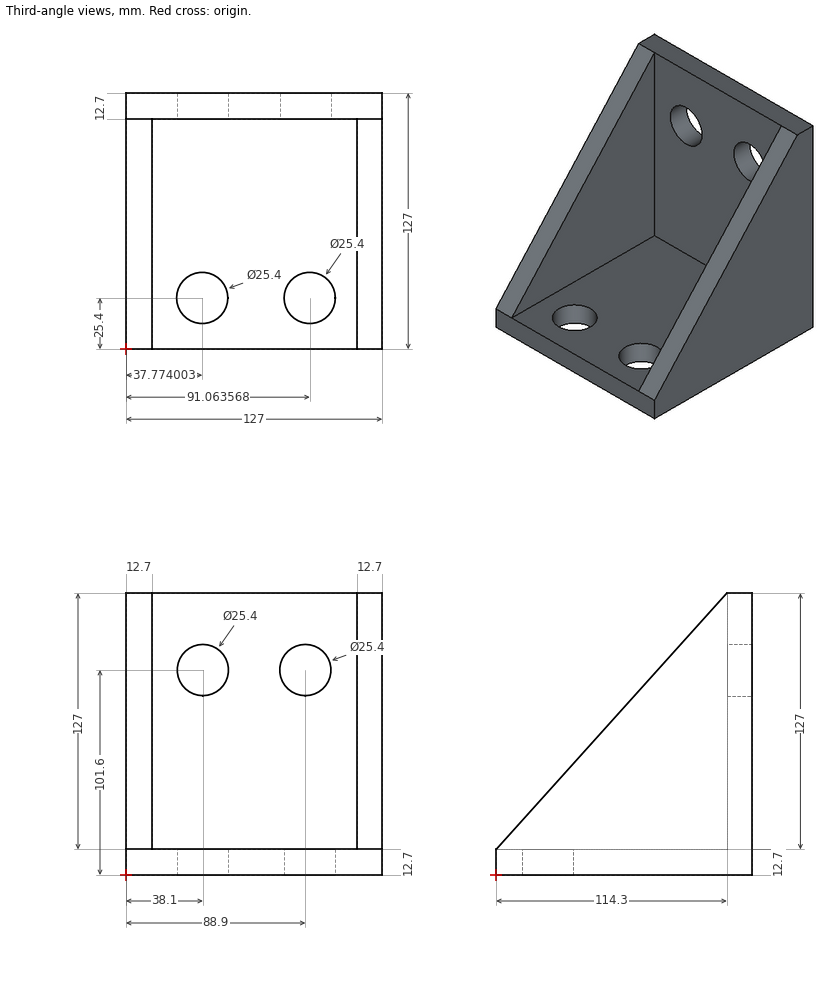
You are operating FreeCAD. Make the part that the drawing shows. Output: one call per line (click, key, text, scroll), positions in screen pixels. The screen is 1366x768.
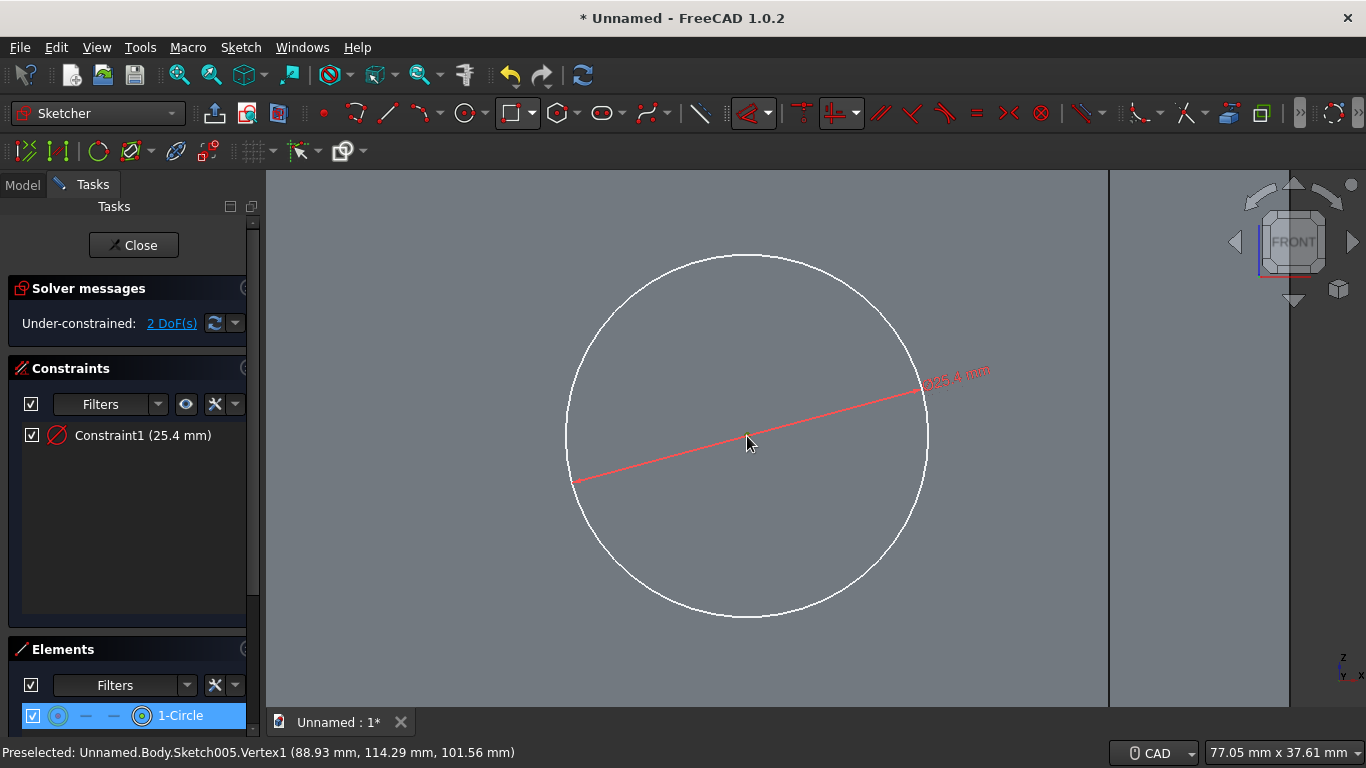
key(l)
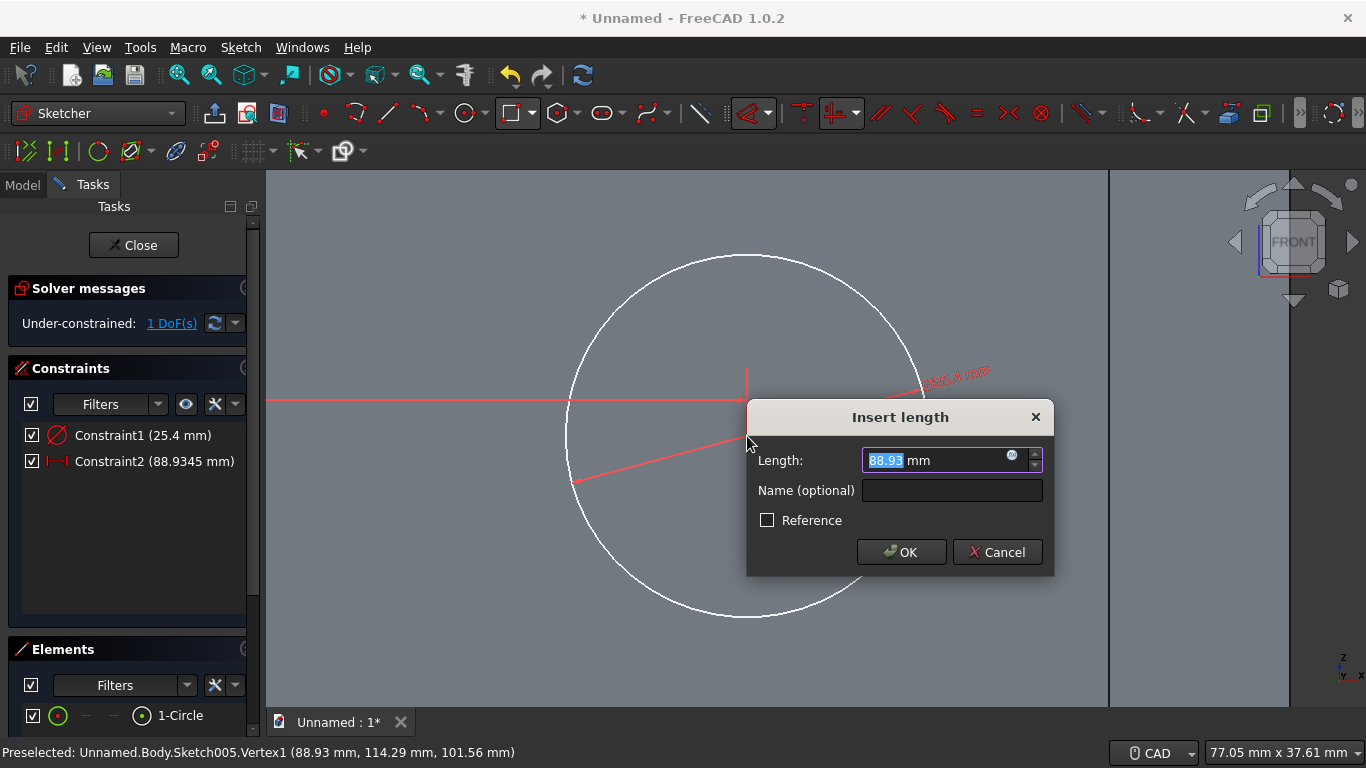
text(88.9)
key(Return)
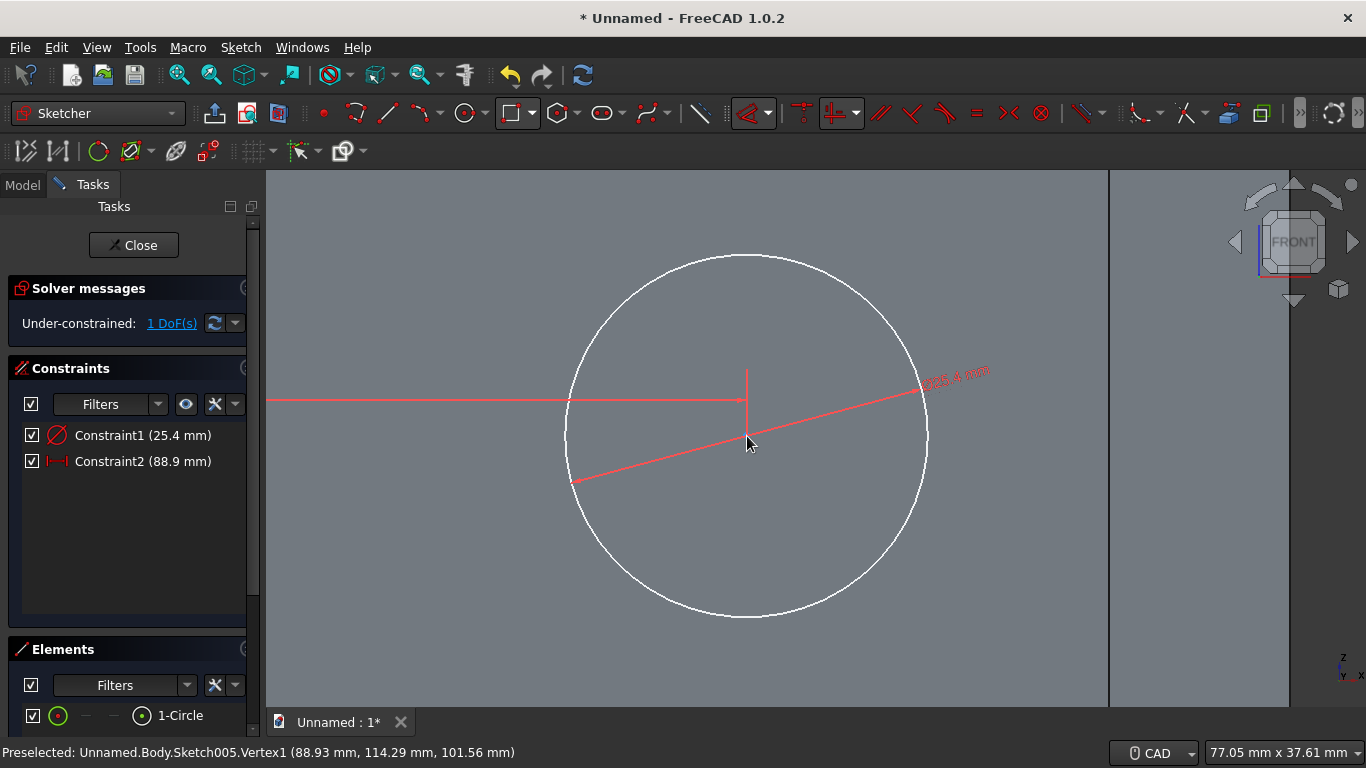
click(747, 436)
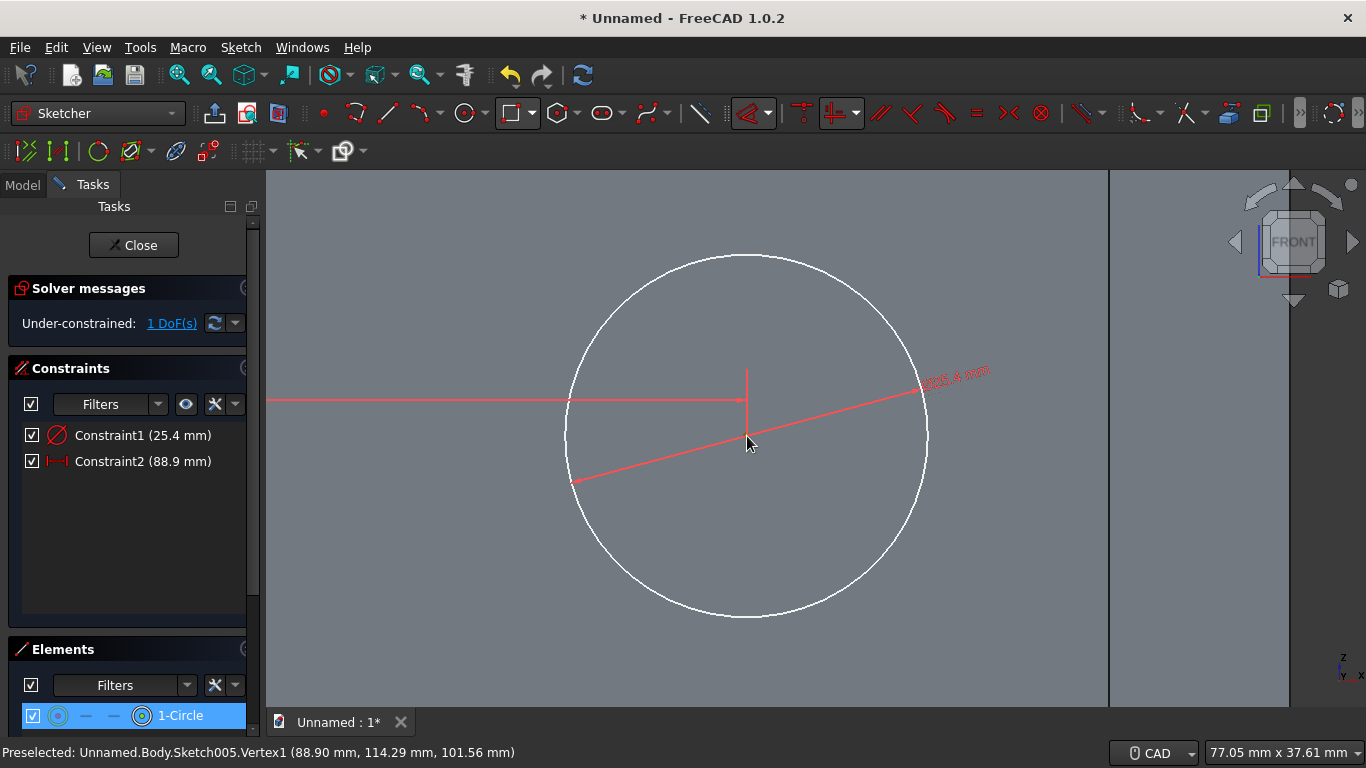
key(i)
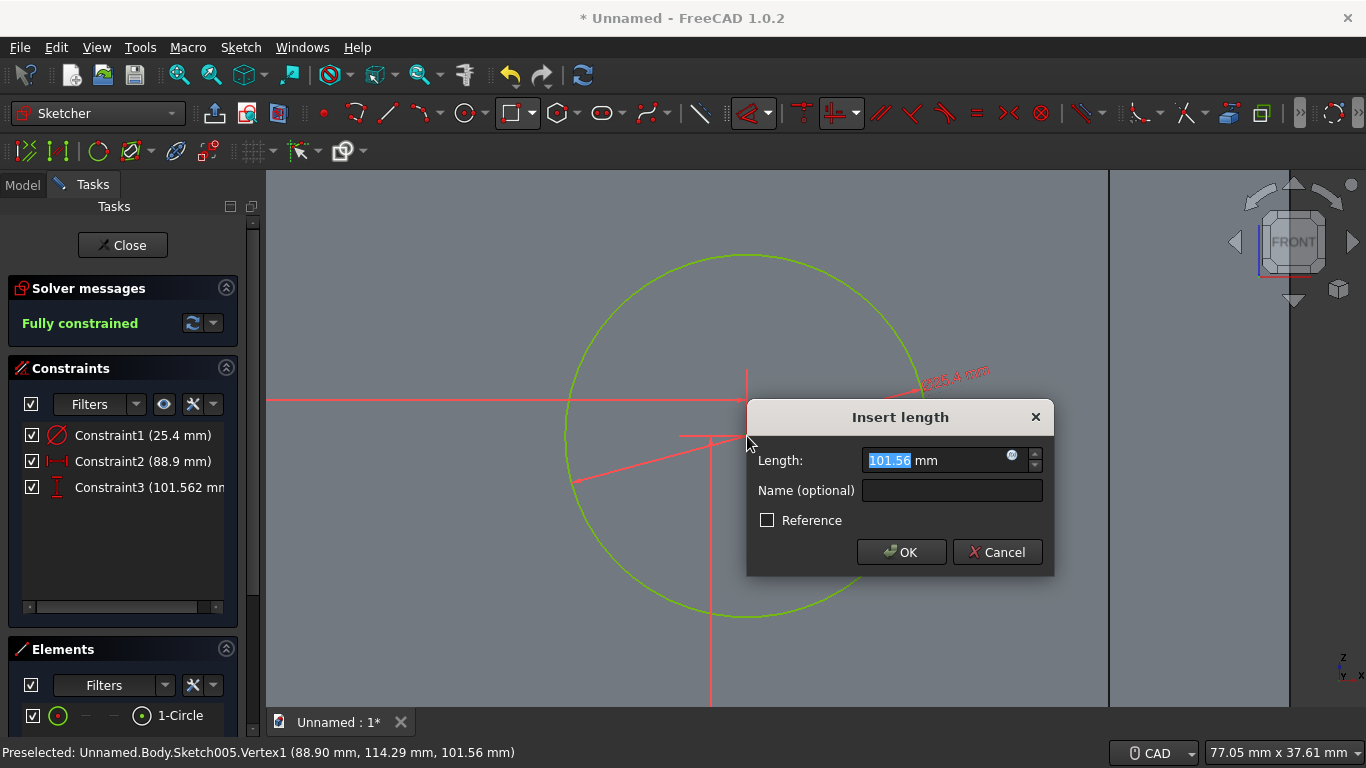
text(101.6)
key(Return)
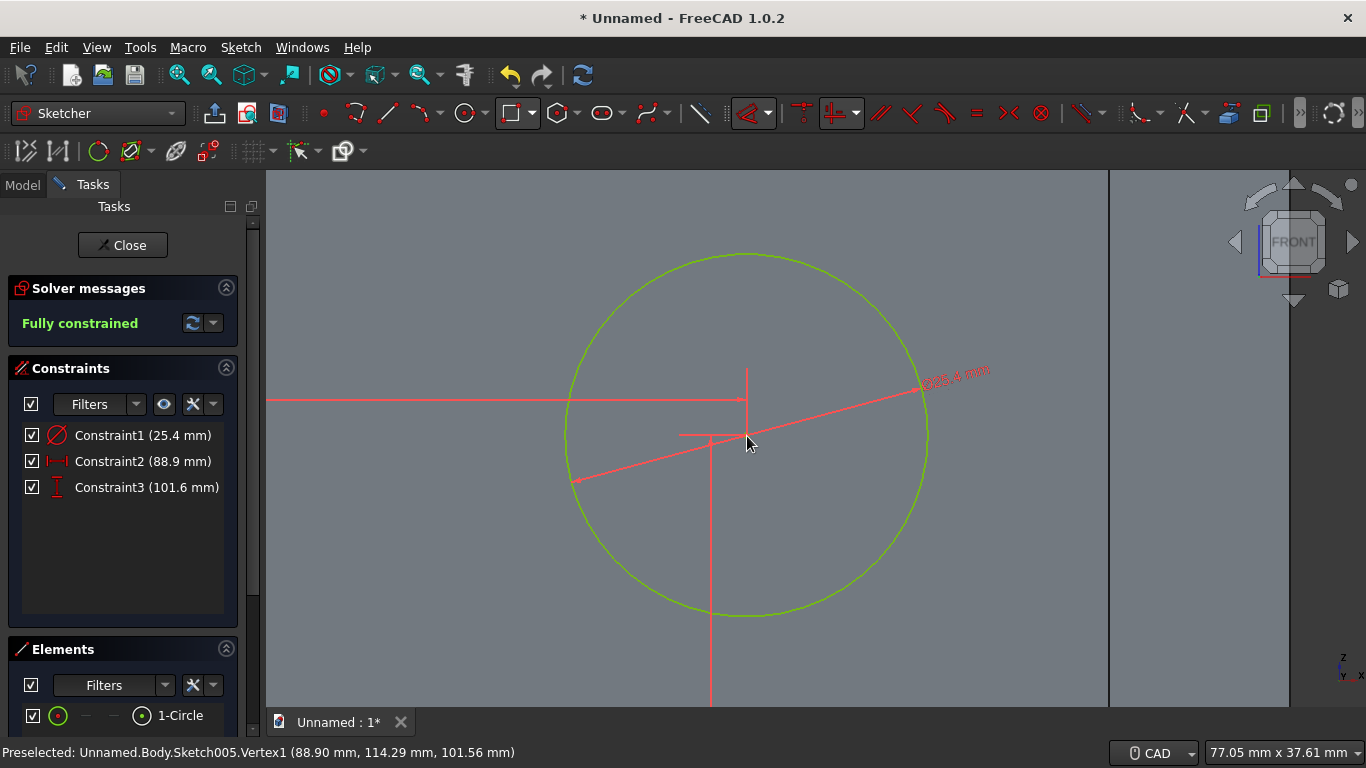
click(123, 245)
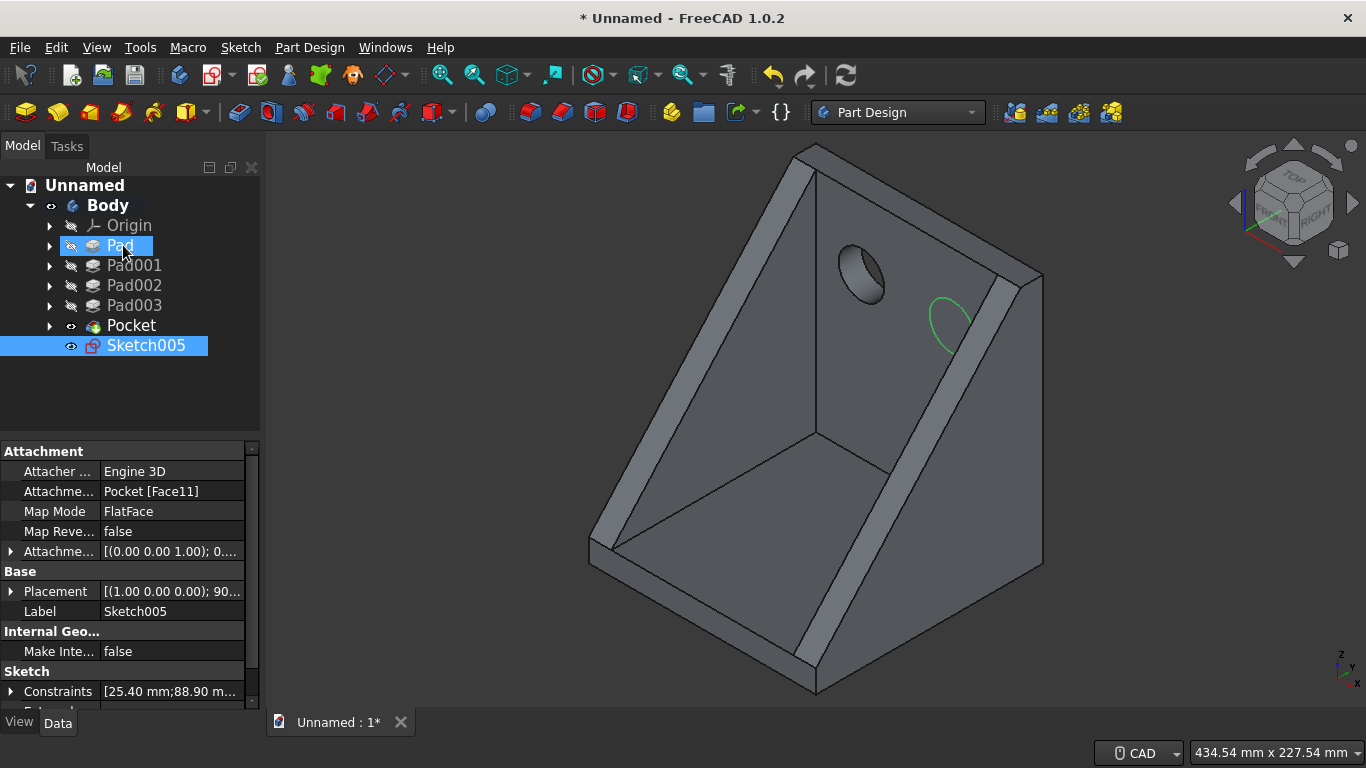
click(240, 112)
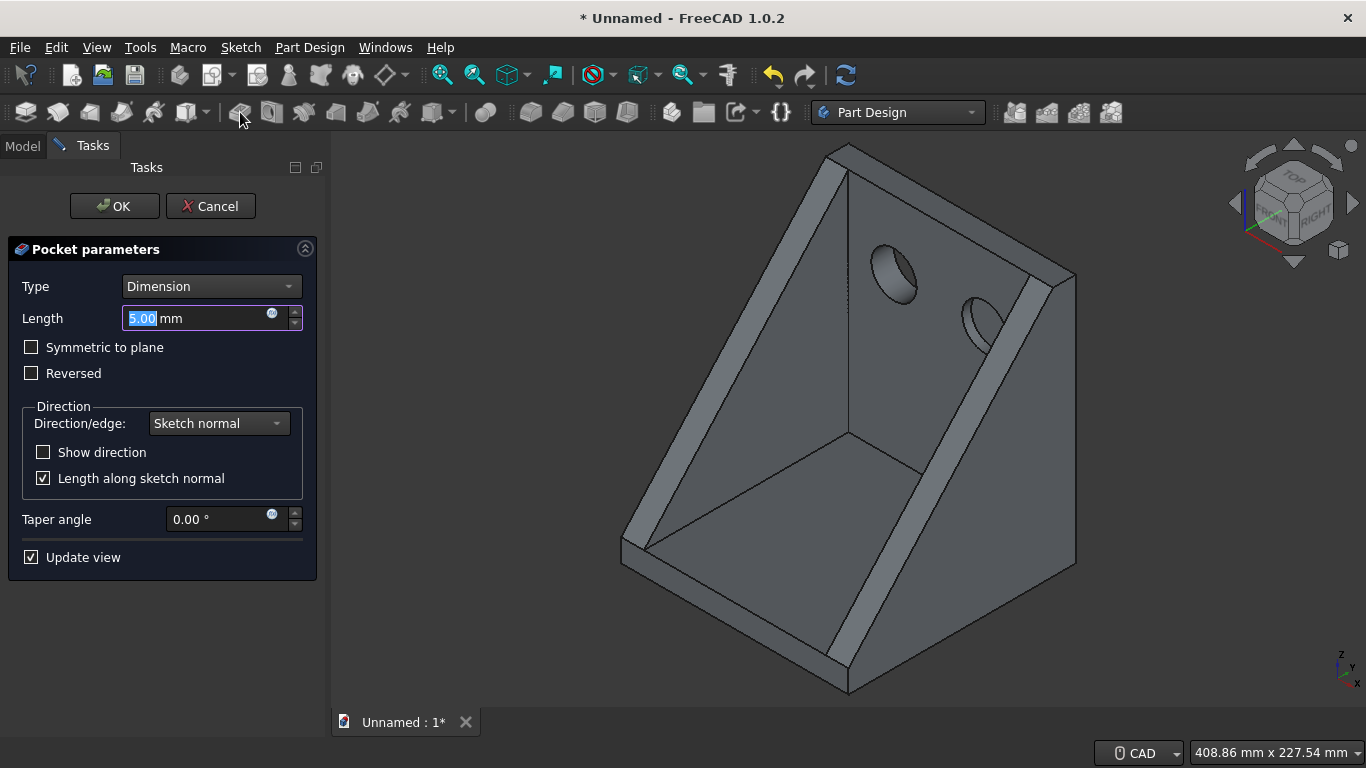
text(12.7)
key(Tab)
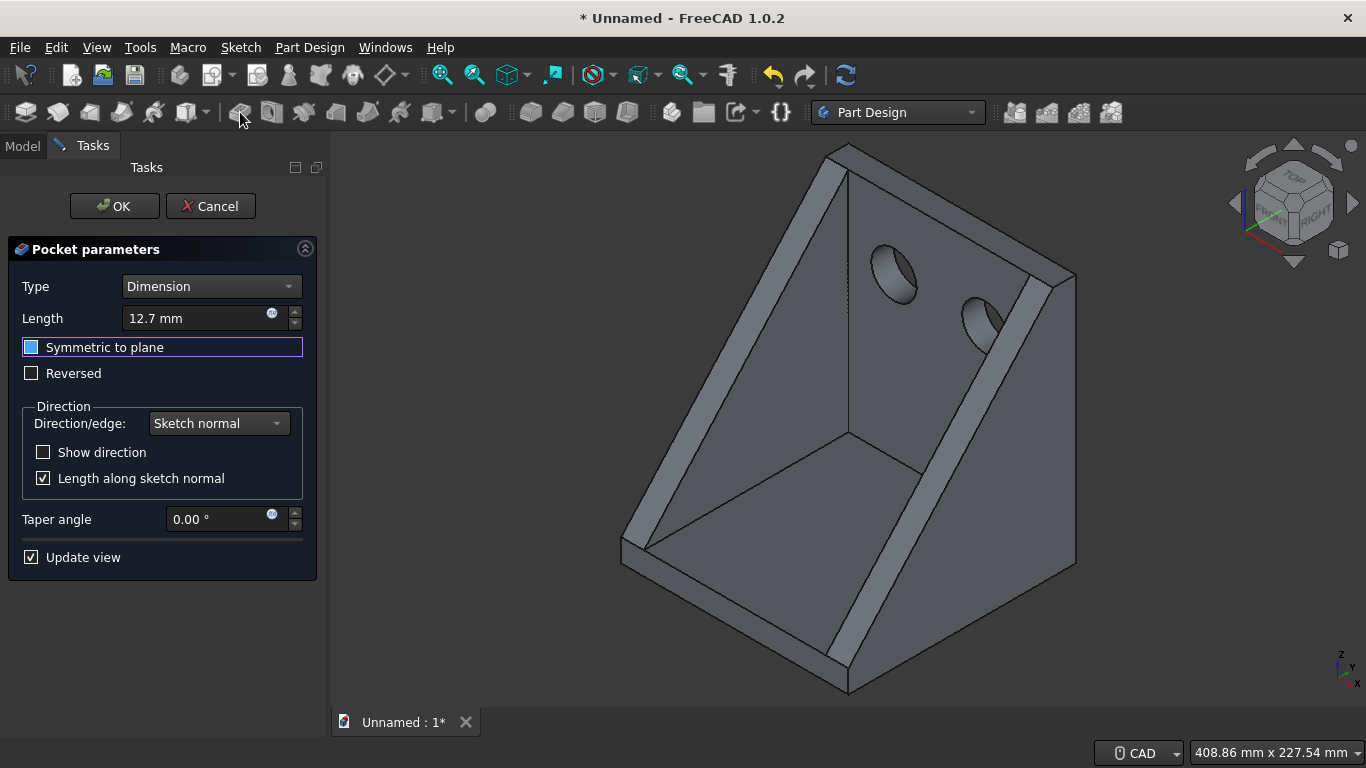
click(115, 206)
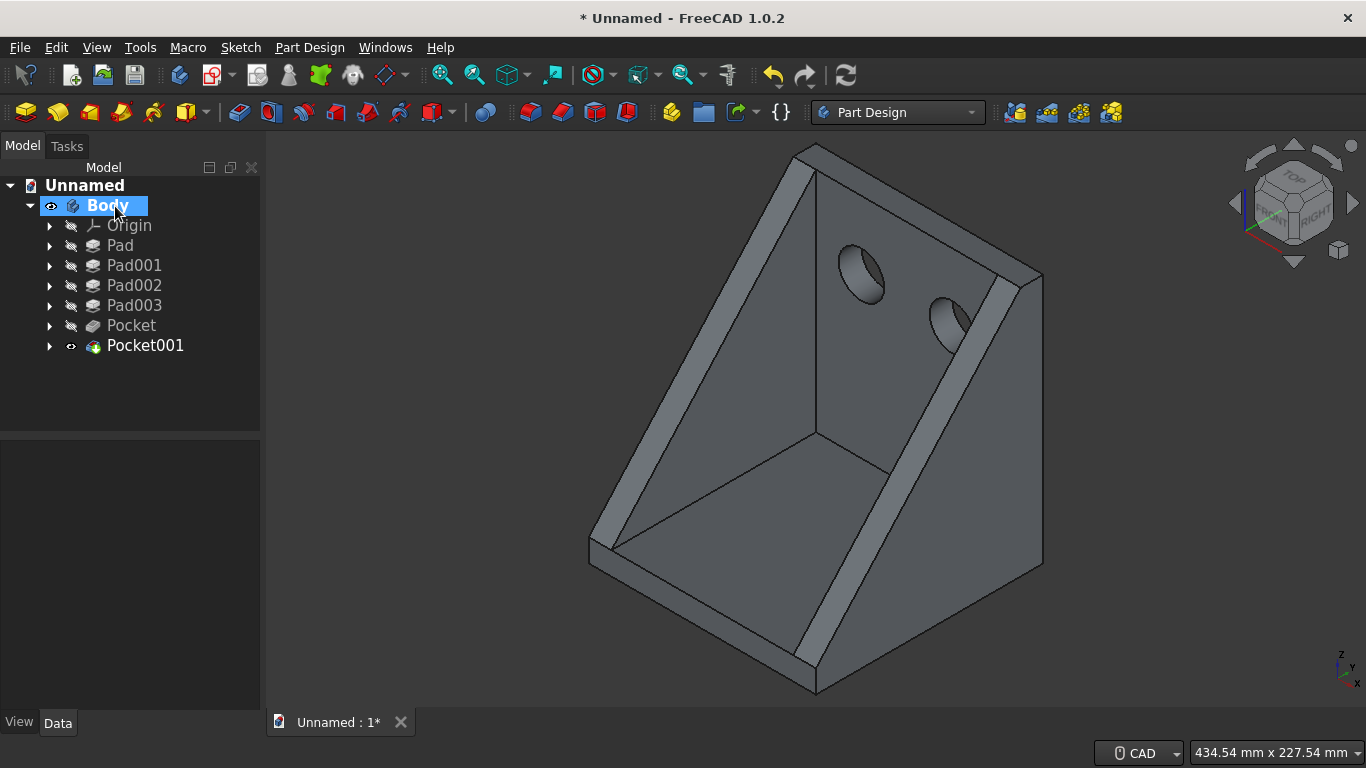
click(805, 543)